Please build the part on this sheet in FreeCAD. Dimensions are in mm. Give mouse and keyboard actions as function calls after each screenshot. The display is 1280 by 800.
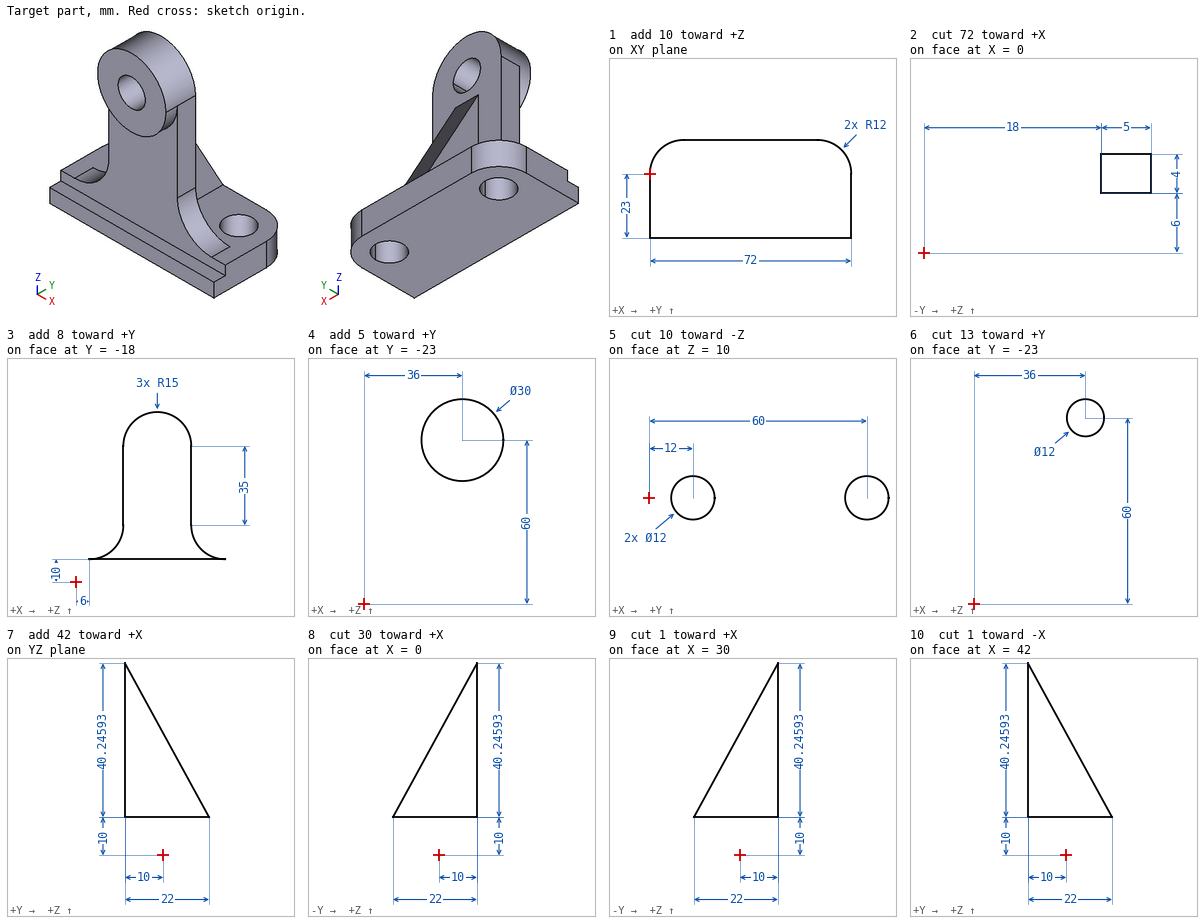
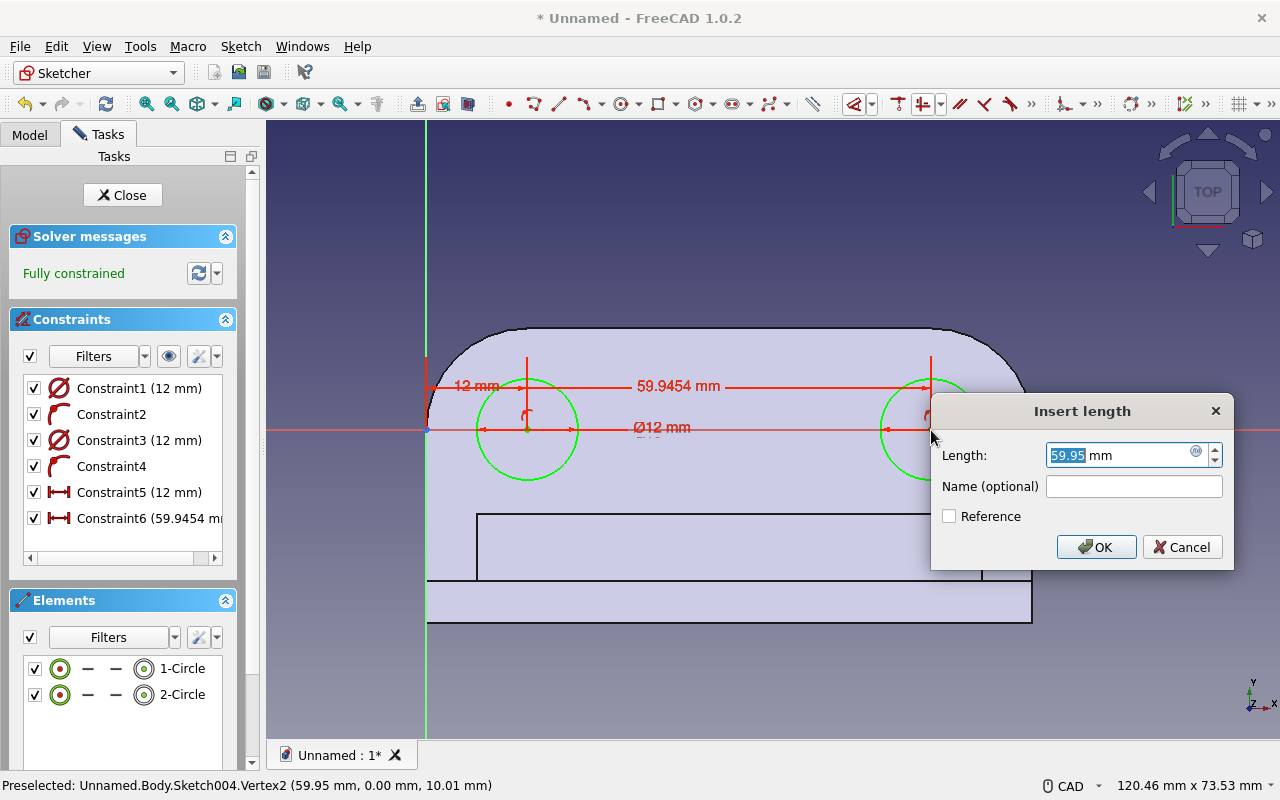
text(60)
key(Return)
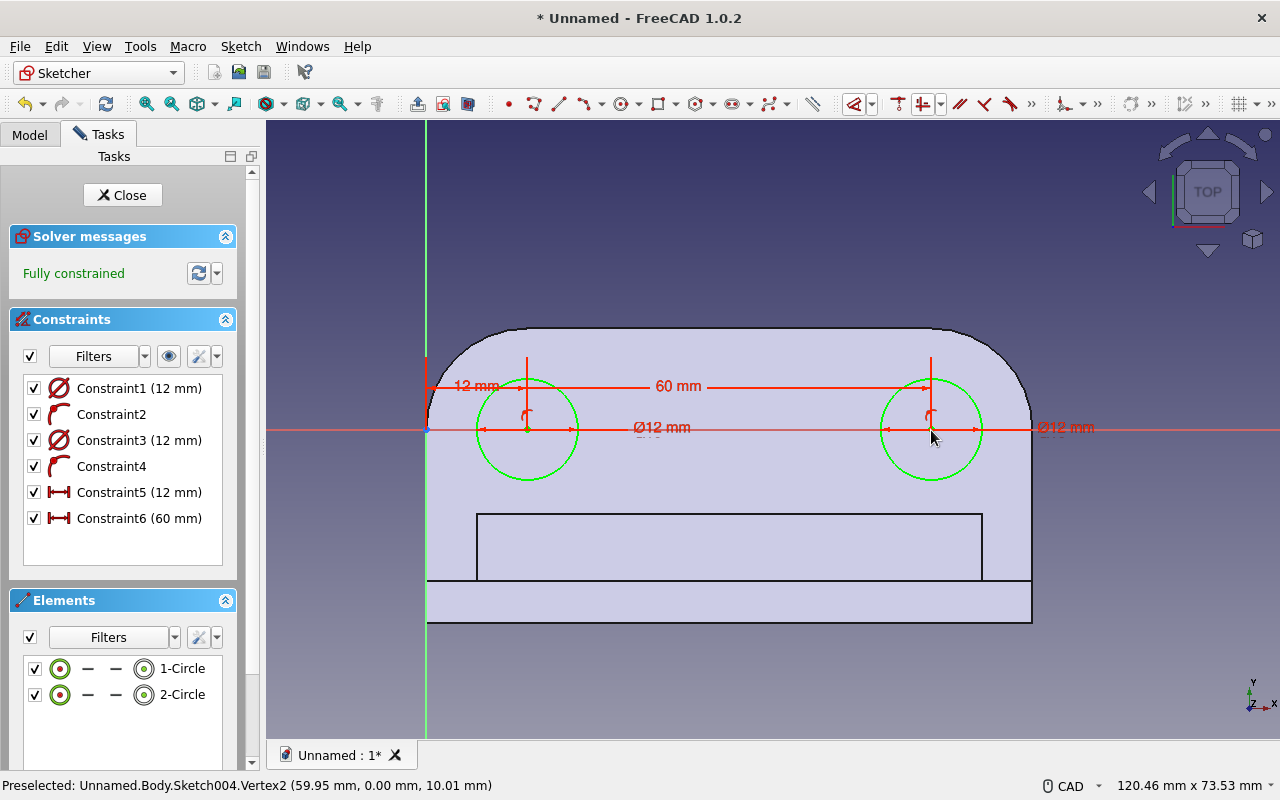
click(123, 195)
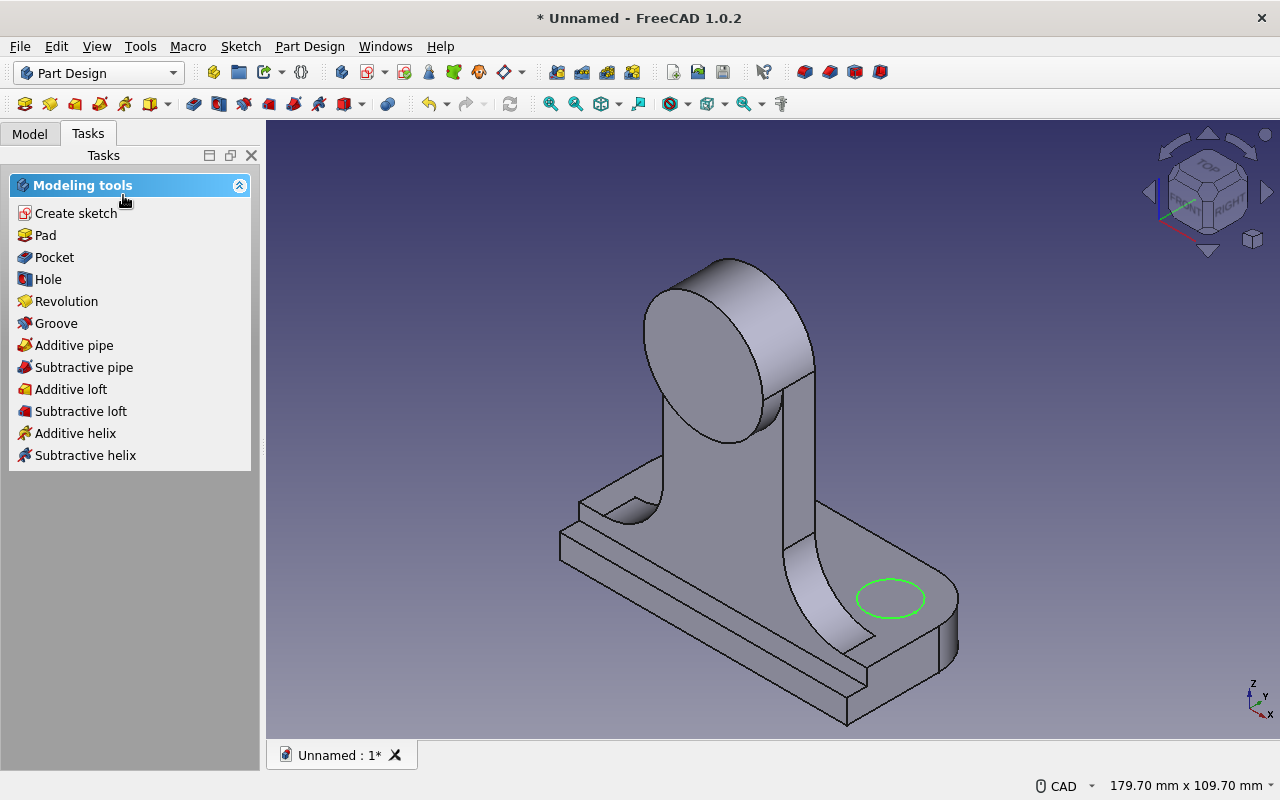
click(194, 104)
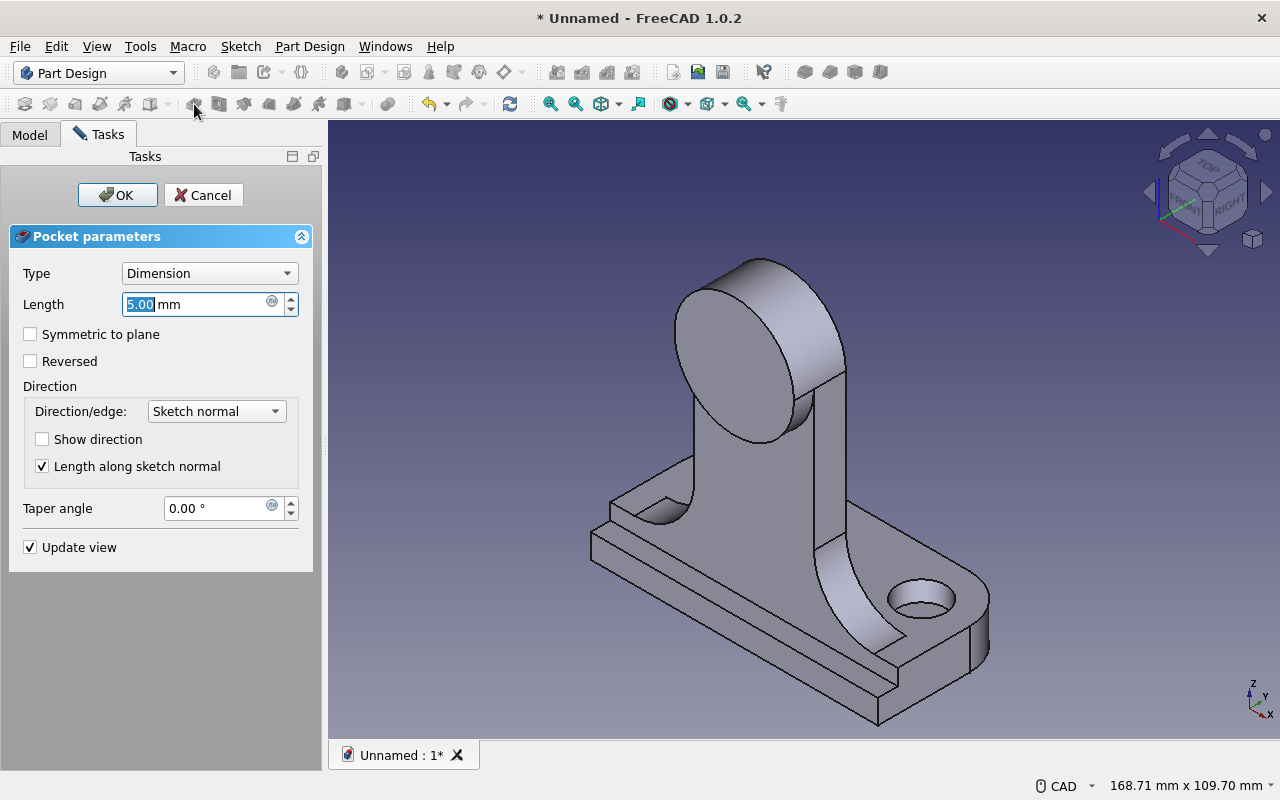
text(10)
key(Tab)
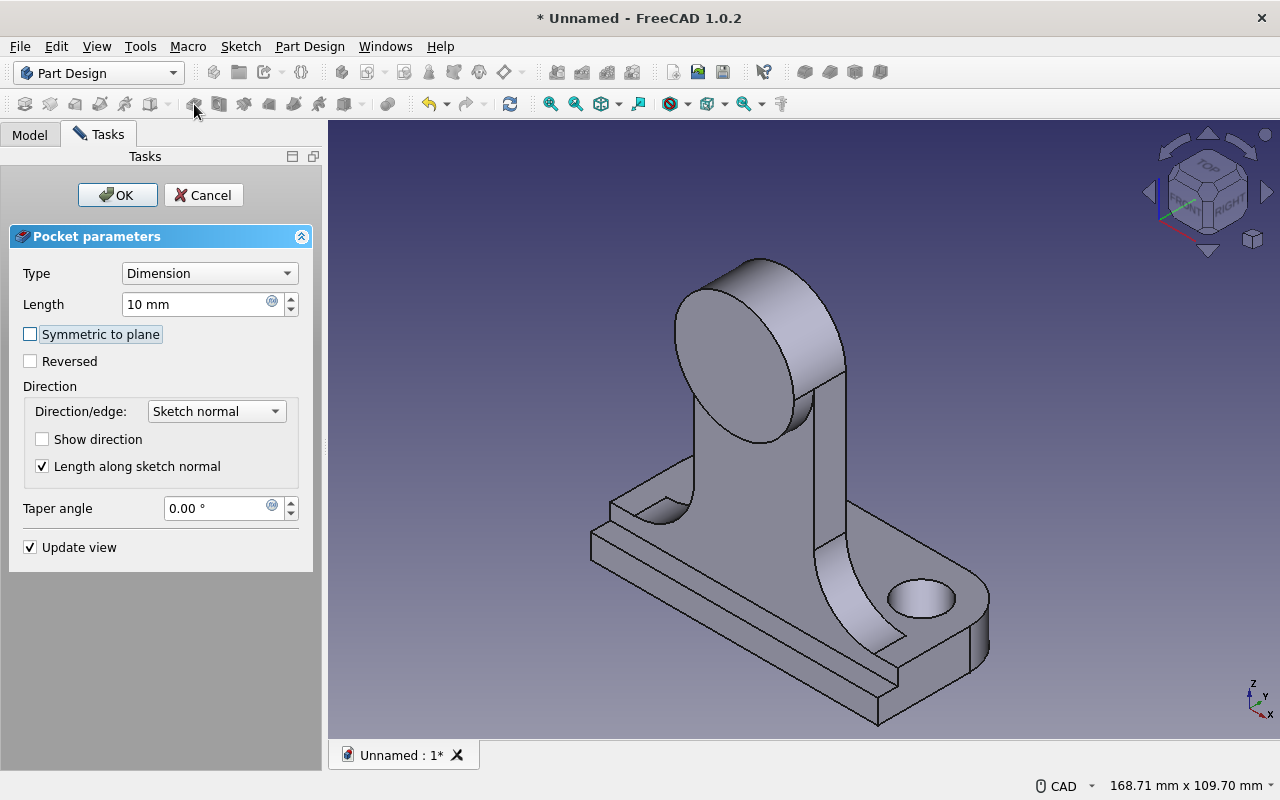
click(118, 195)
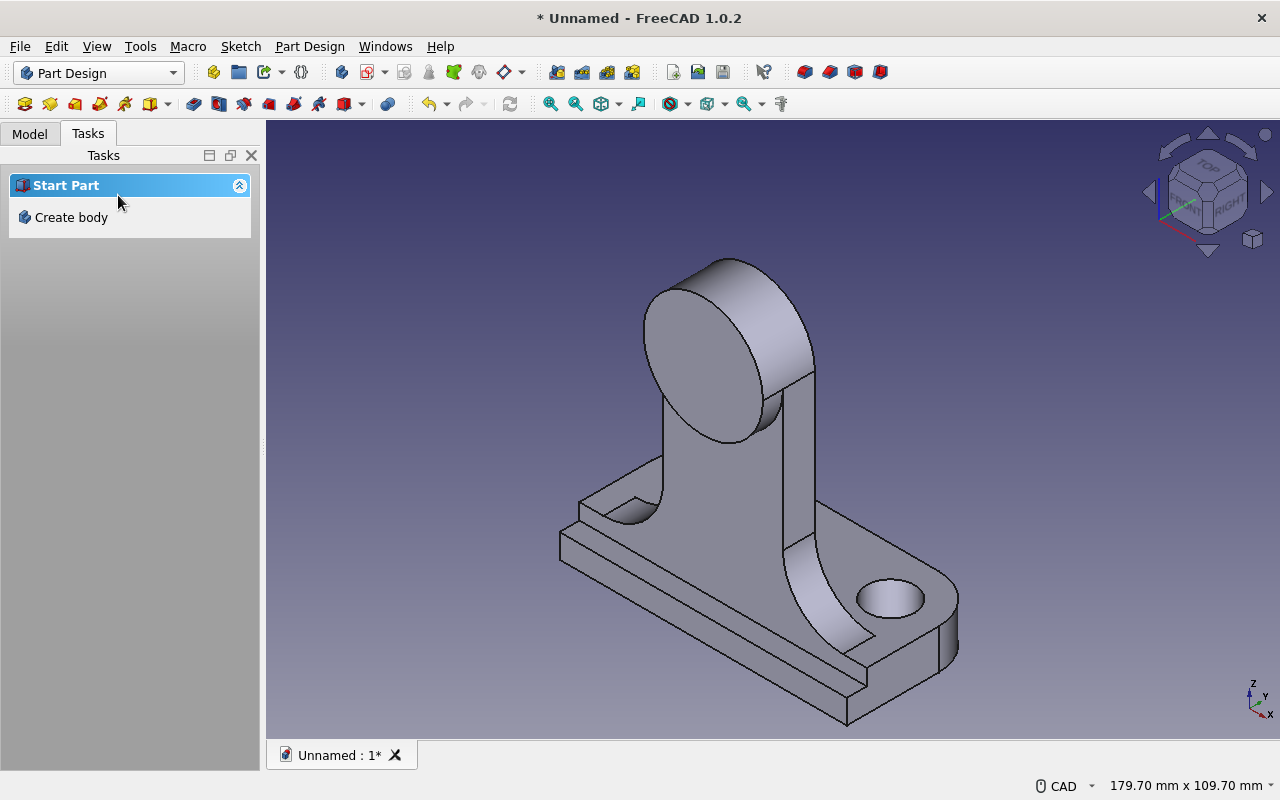
click(703, 365)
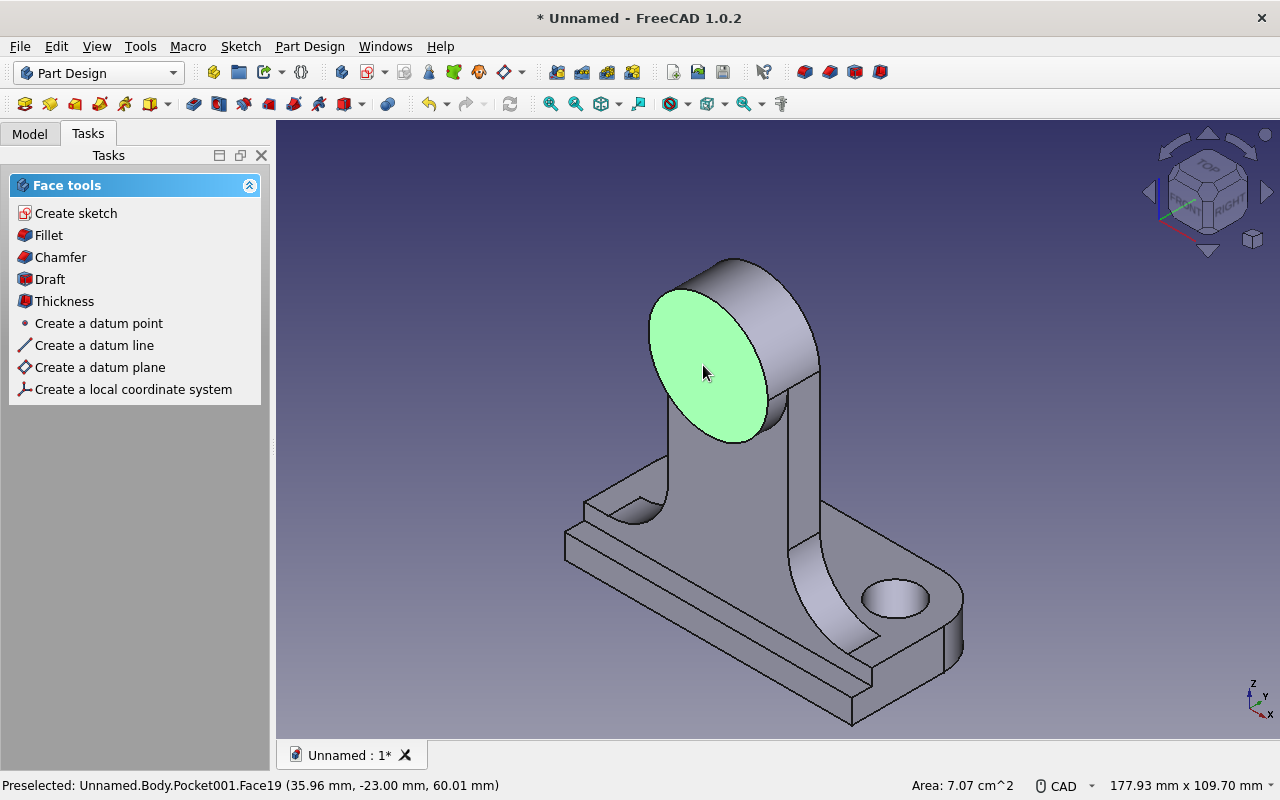
click(366, 72)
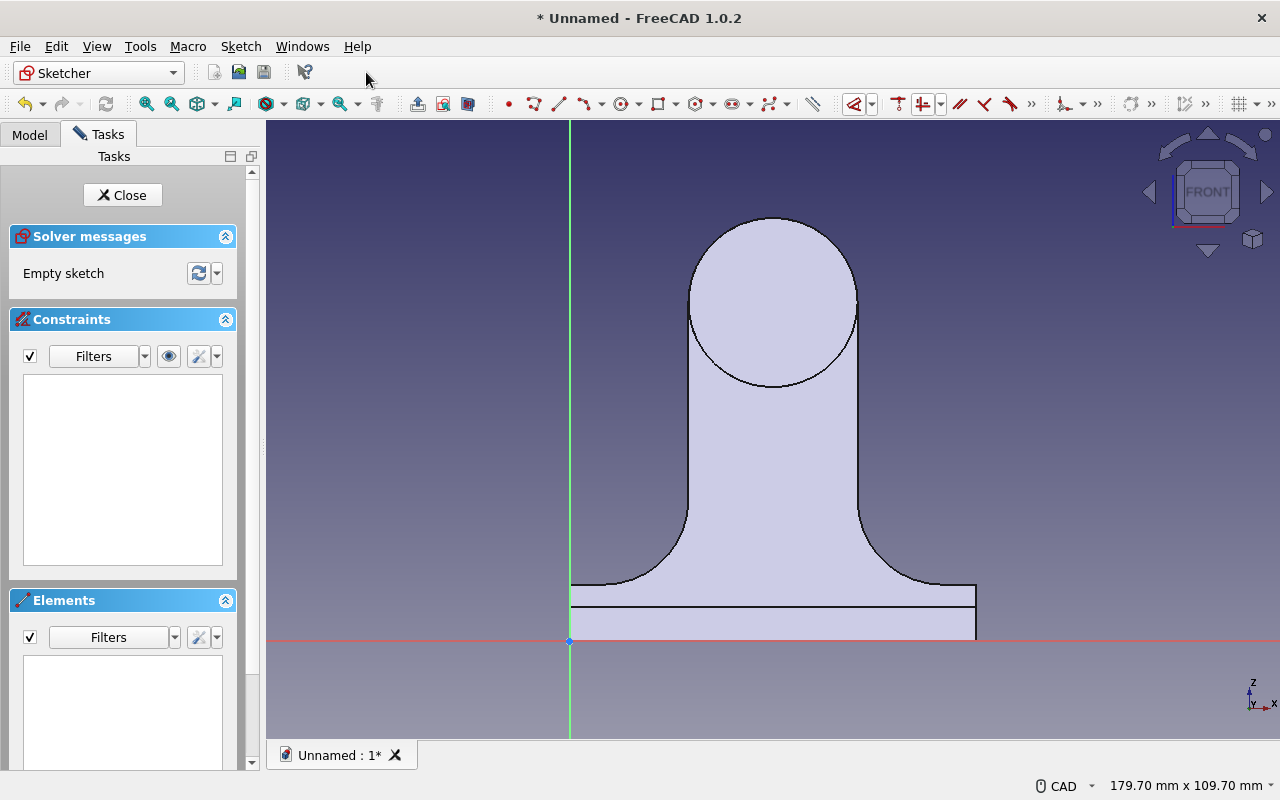
scroll(787, 277, up, 9)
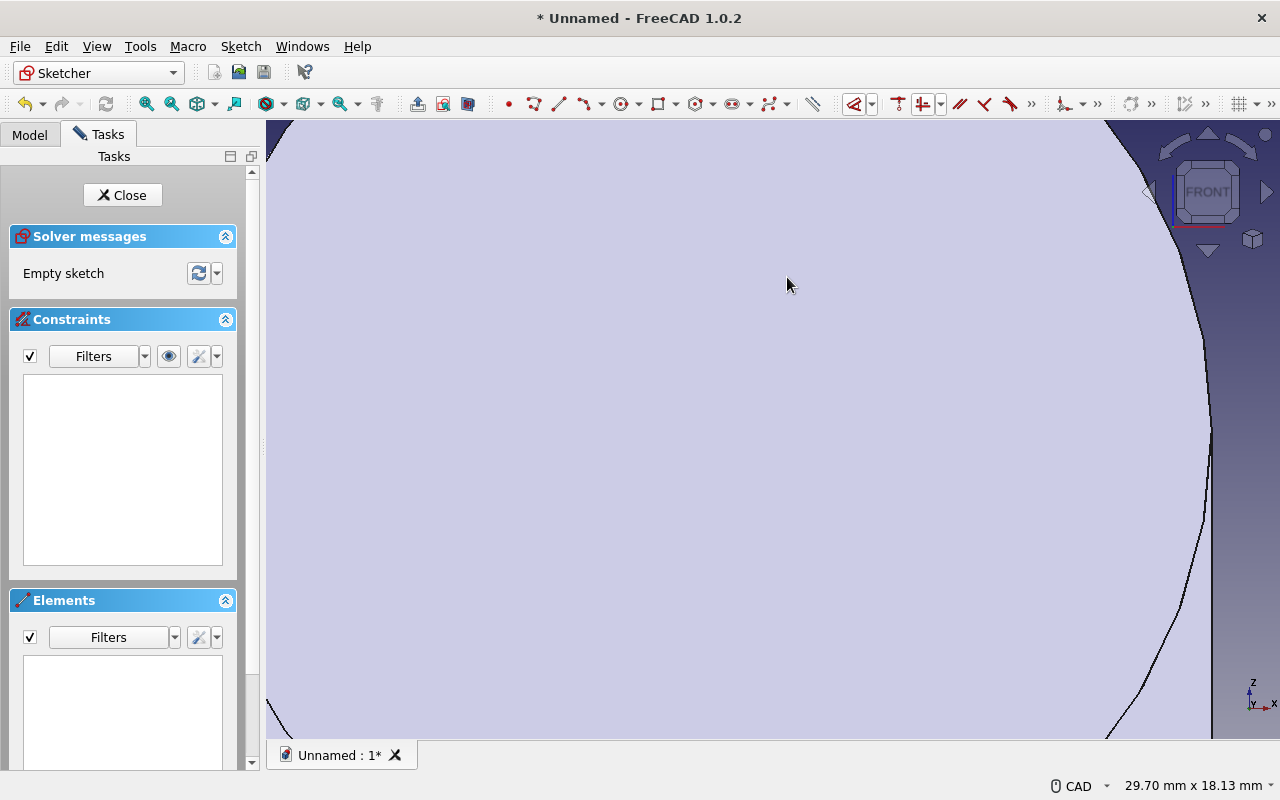
click(620, 104)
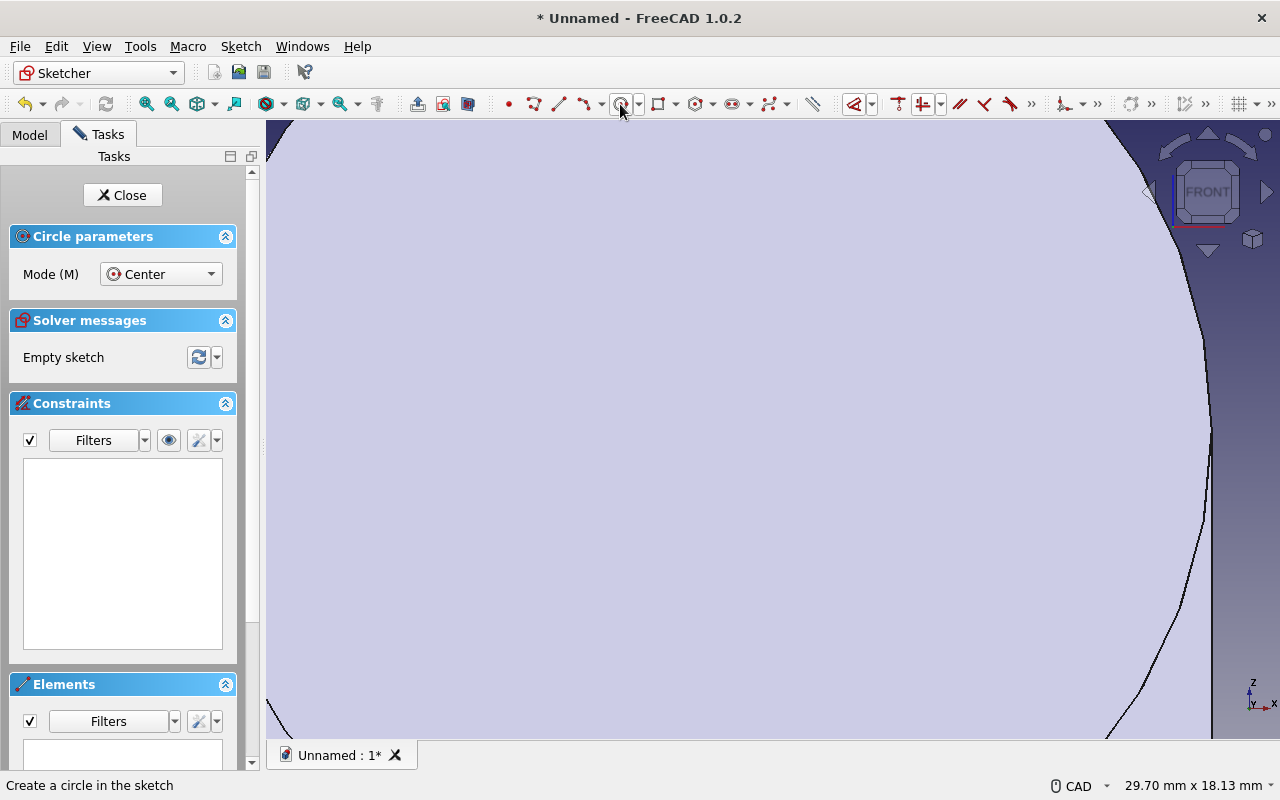
click(700, 430)
move(845, 285)